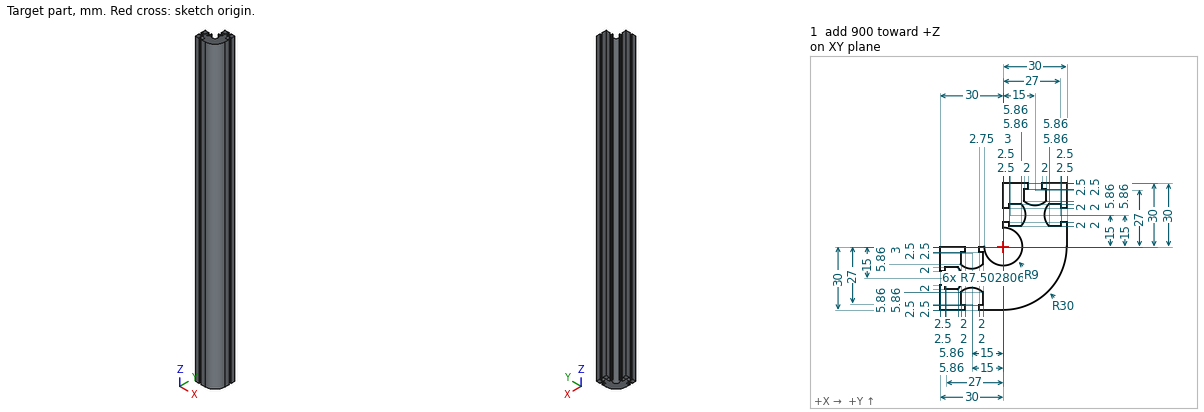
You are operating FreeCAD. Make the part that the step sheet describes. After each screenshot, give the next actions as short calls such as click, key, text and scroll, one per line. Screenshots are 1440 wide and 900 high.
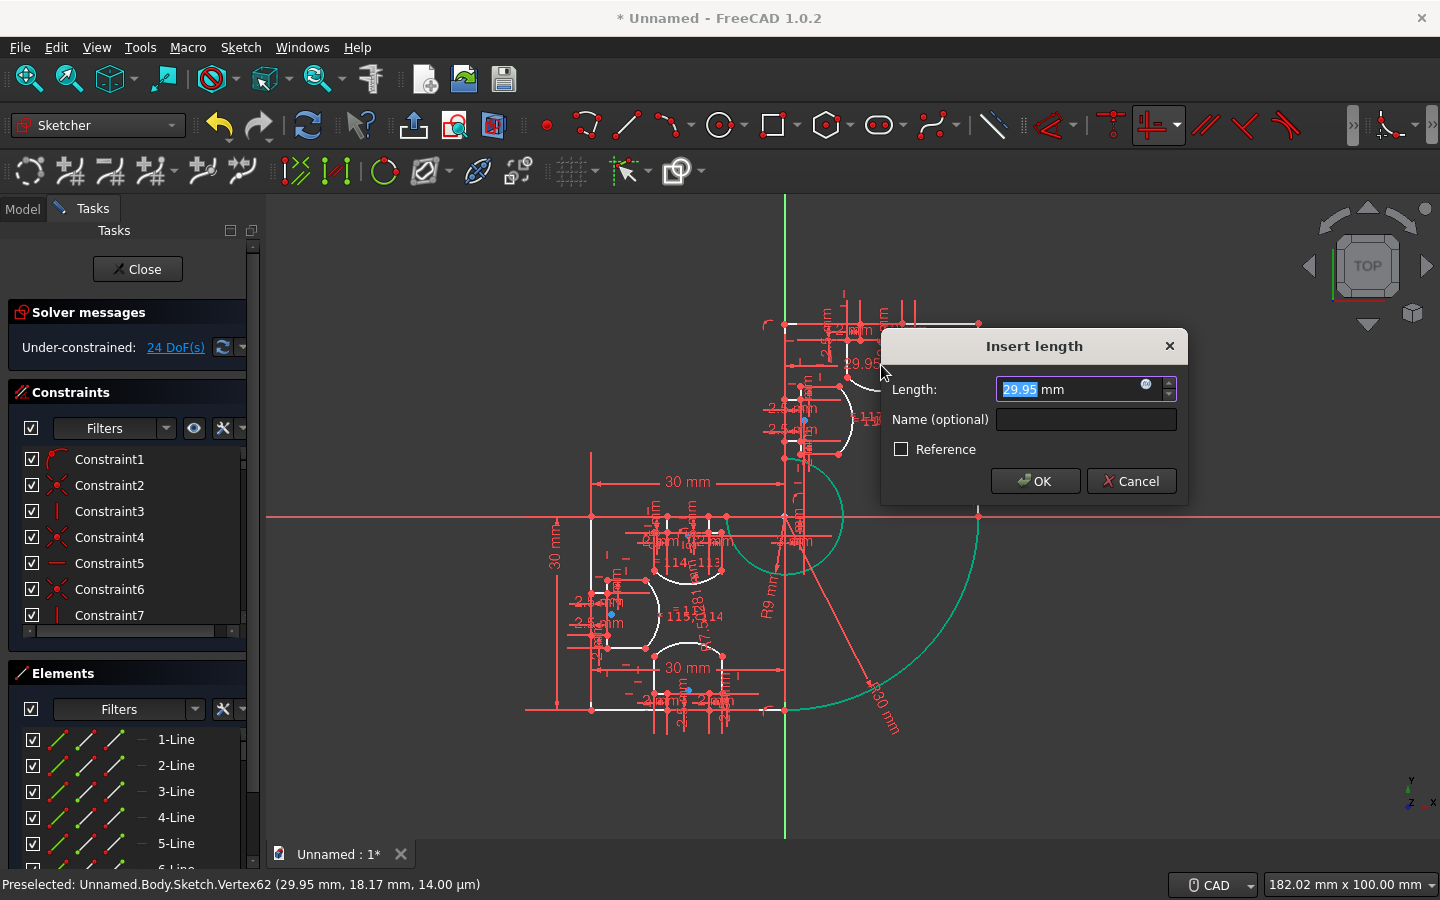
text(30)
key(Return)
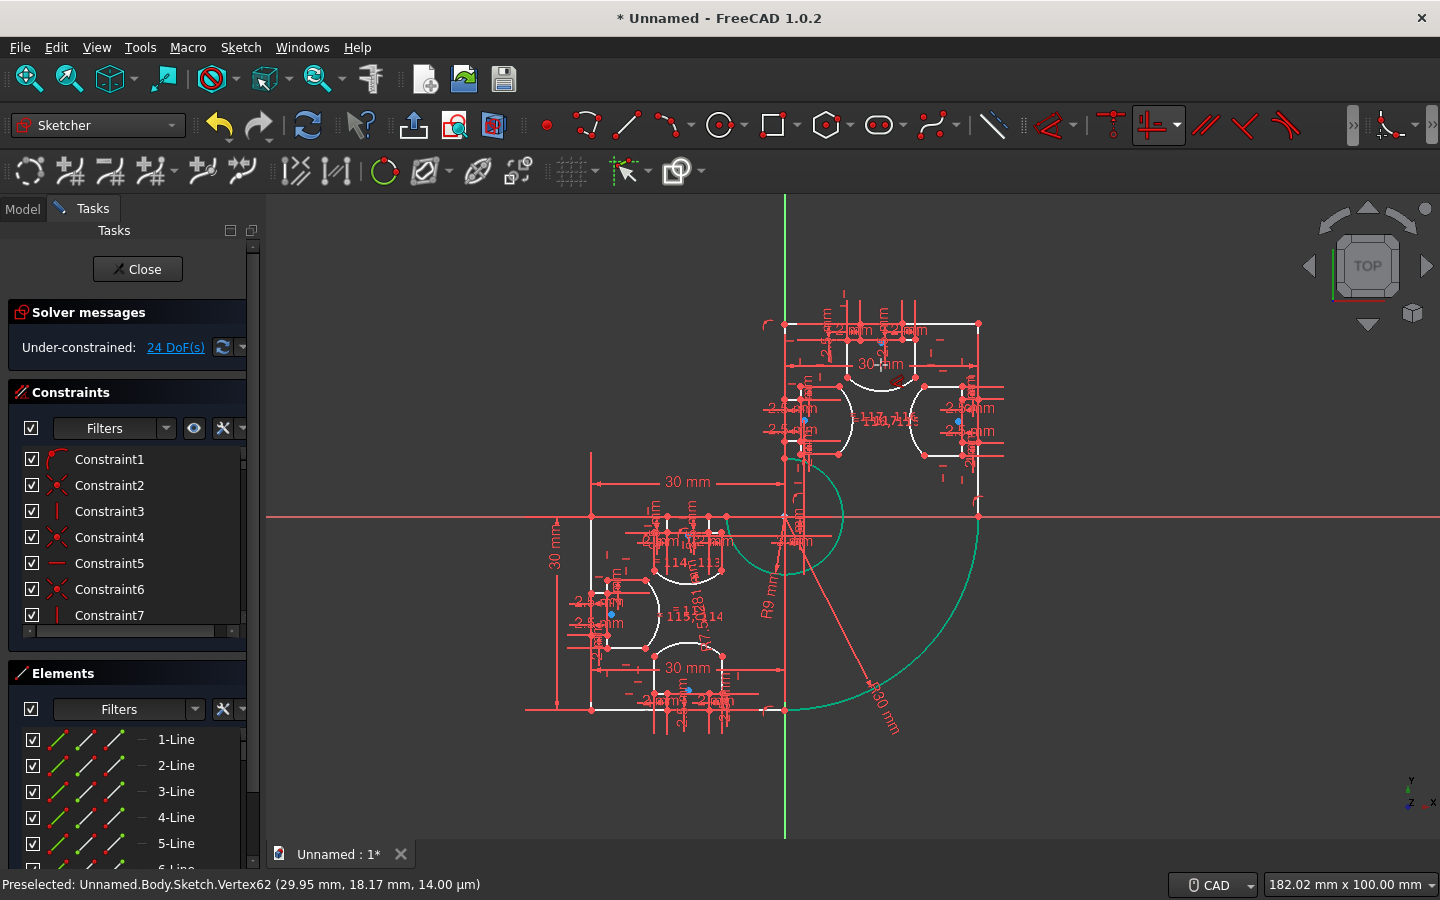
click(978, 324)
click(1012, 353)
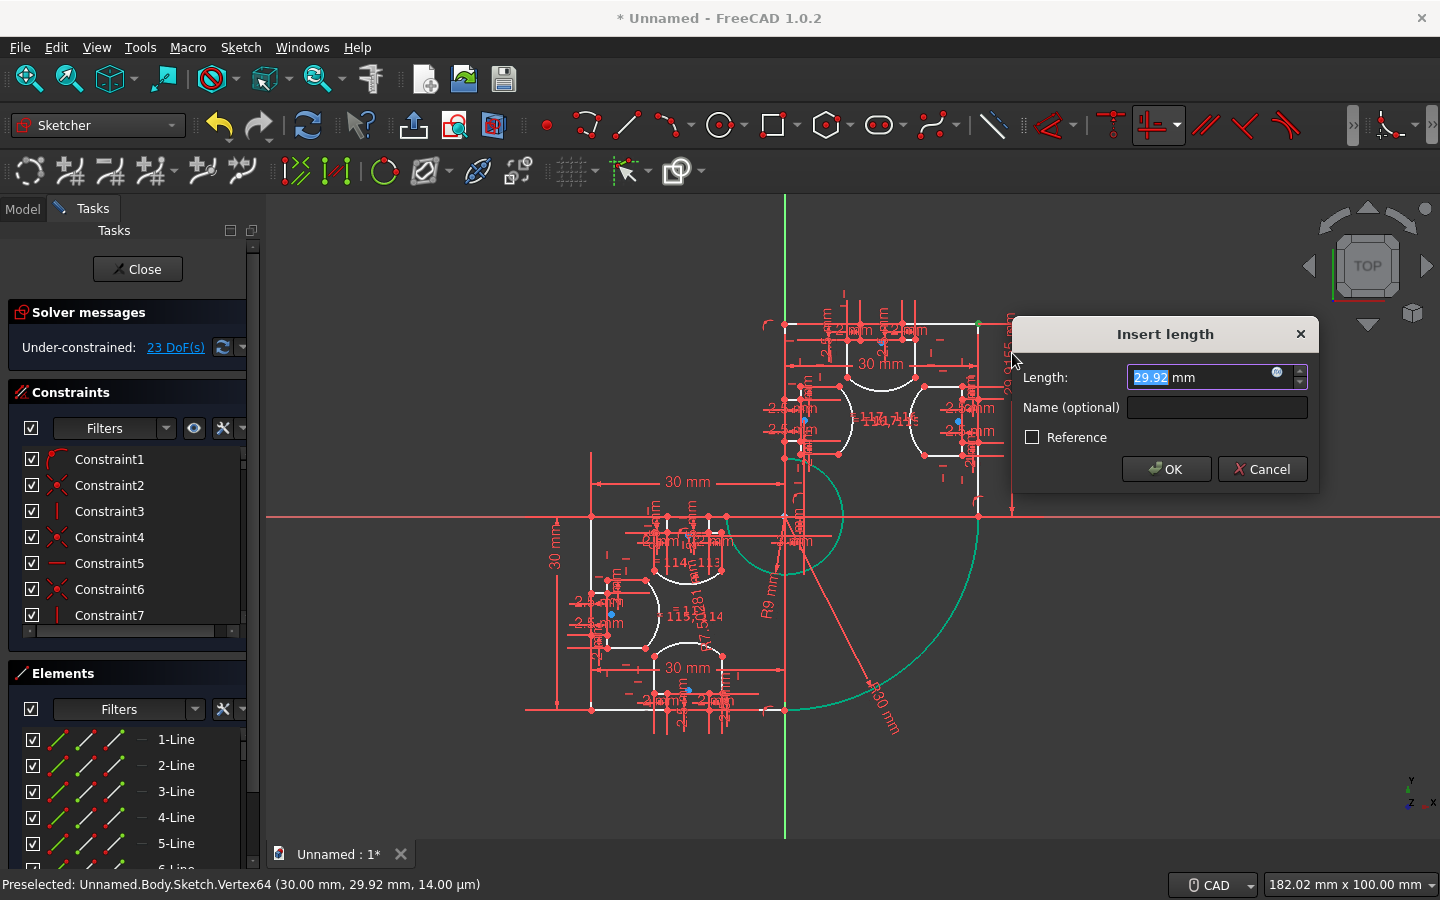
text(30)
key(Return)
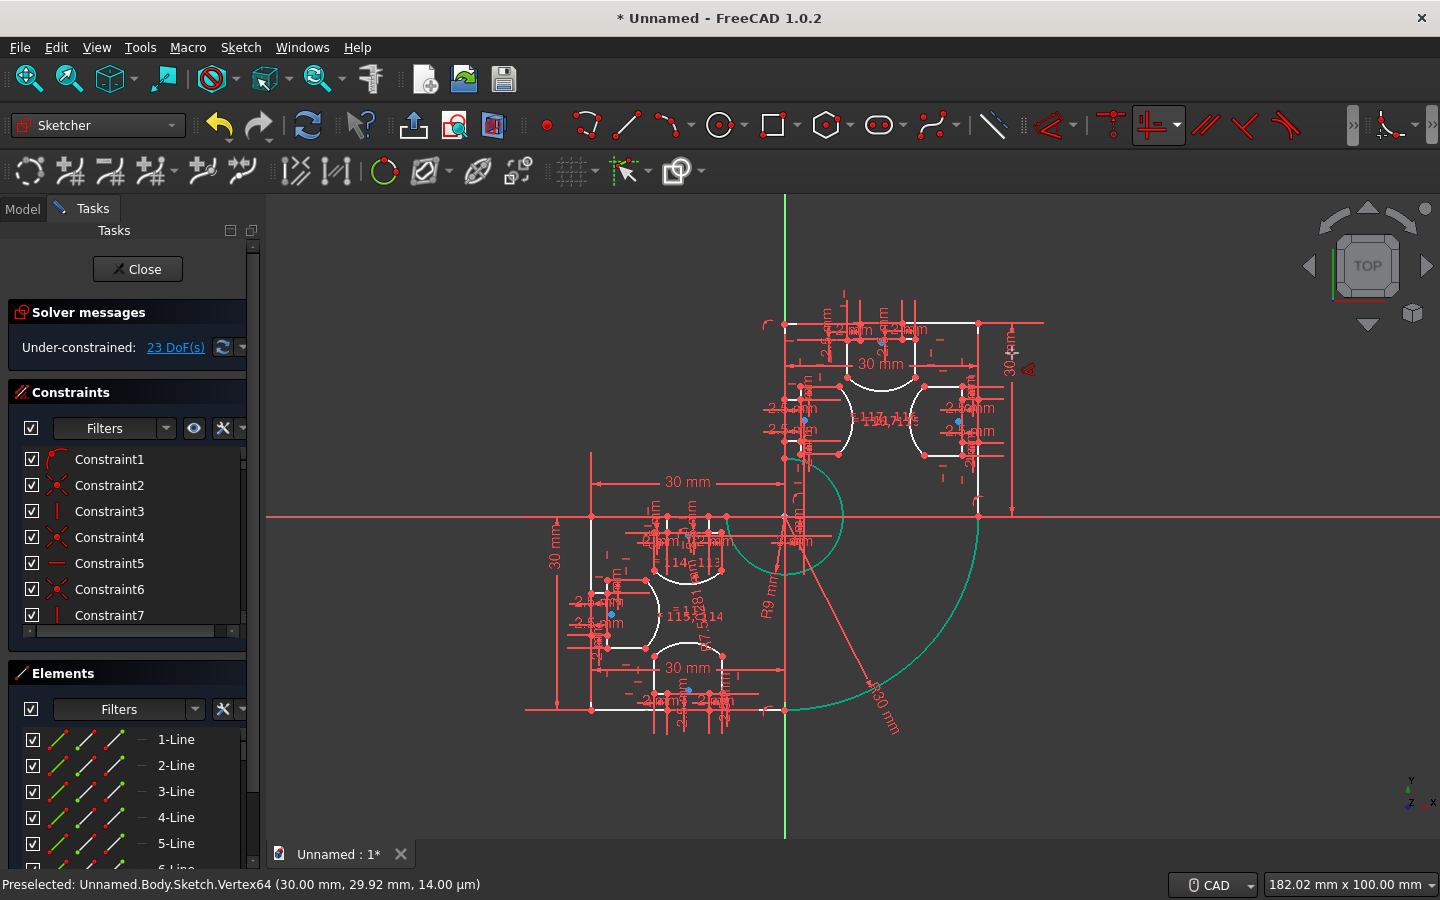
click(860, 324)
click(894, 420)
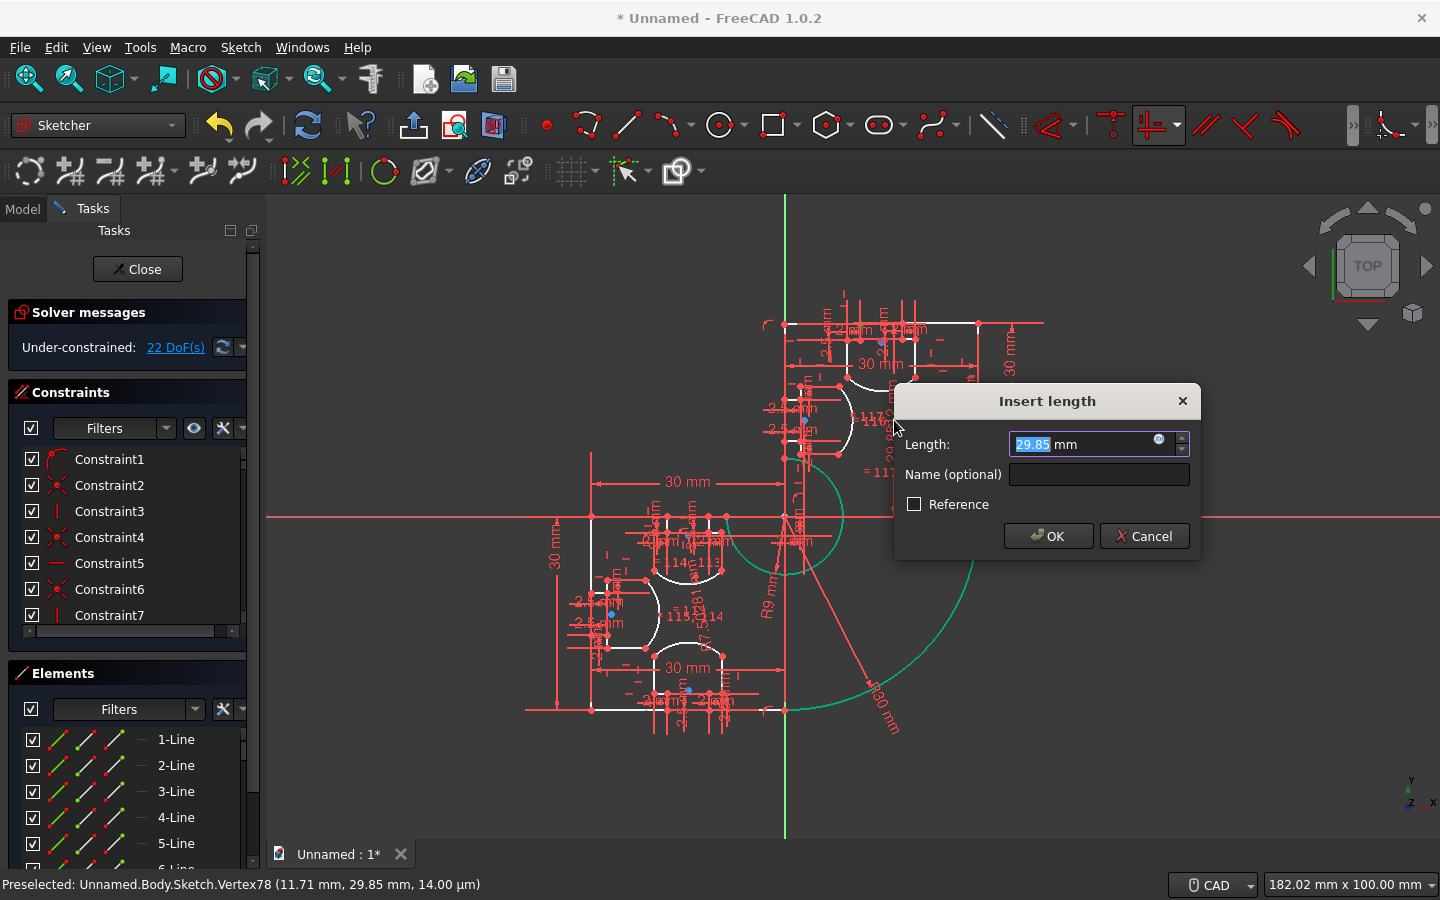
text(30)
key(Return)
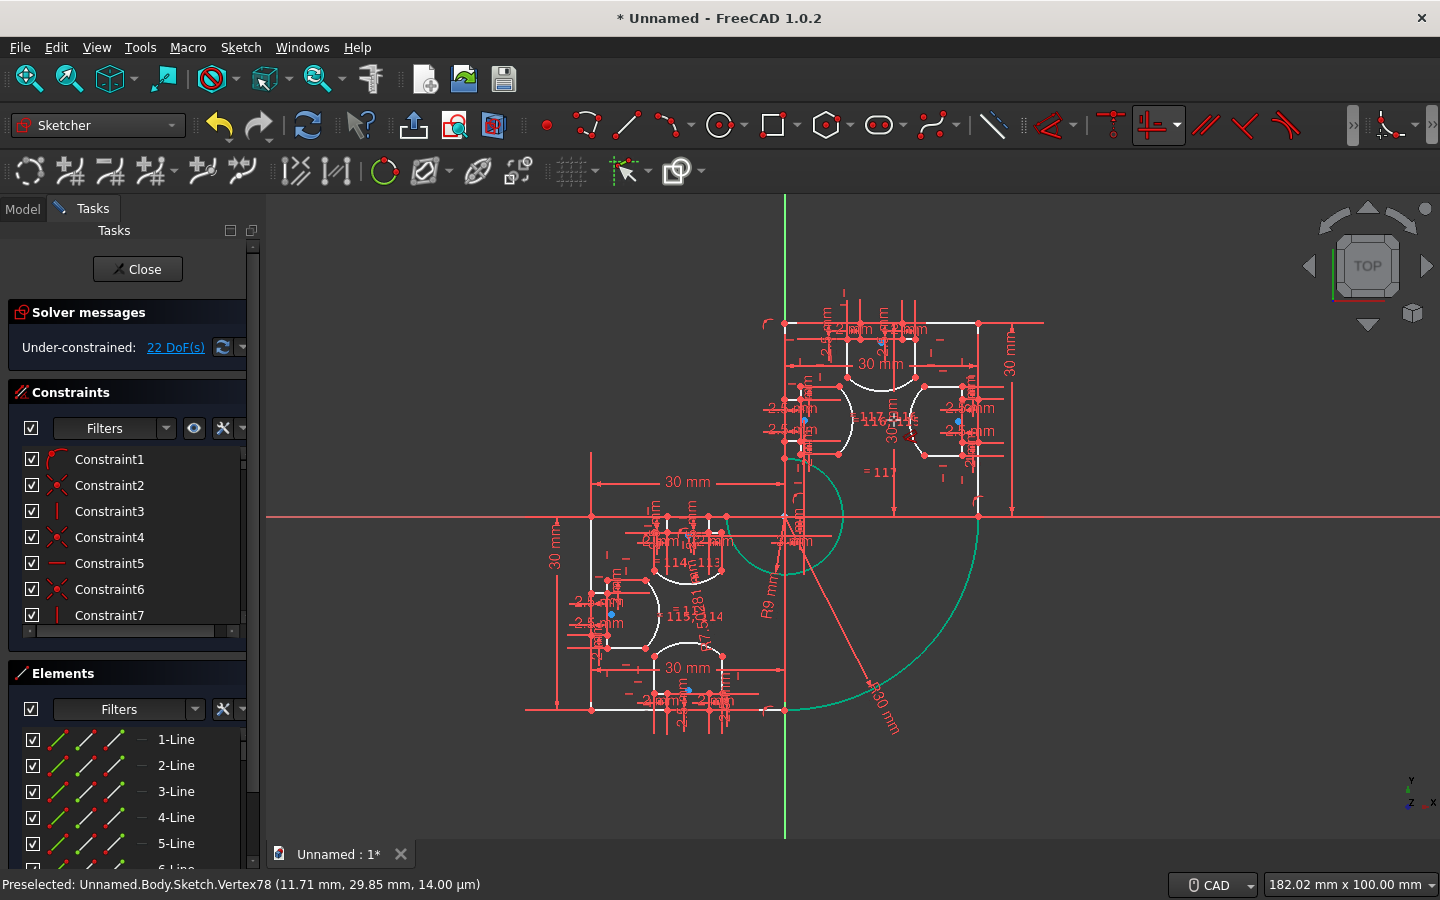
click(688, 536)
click(736, 570)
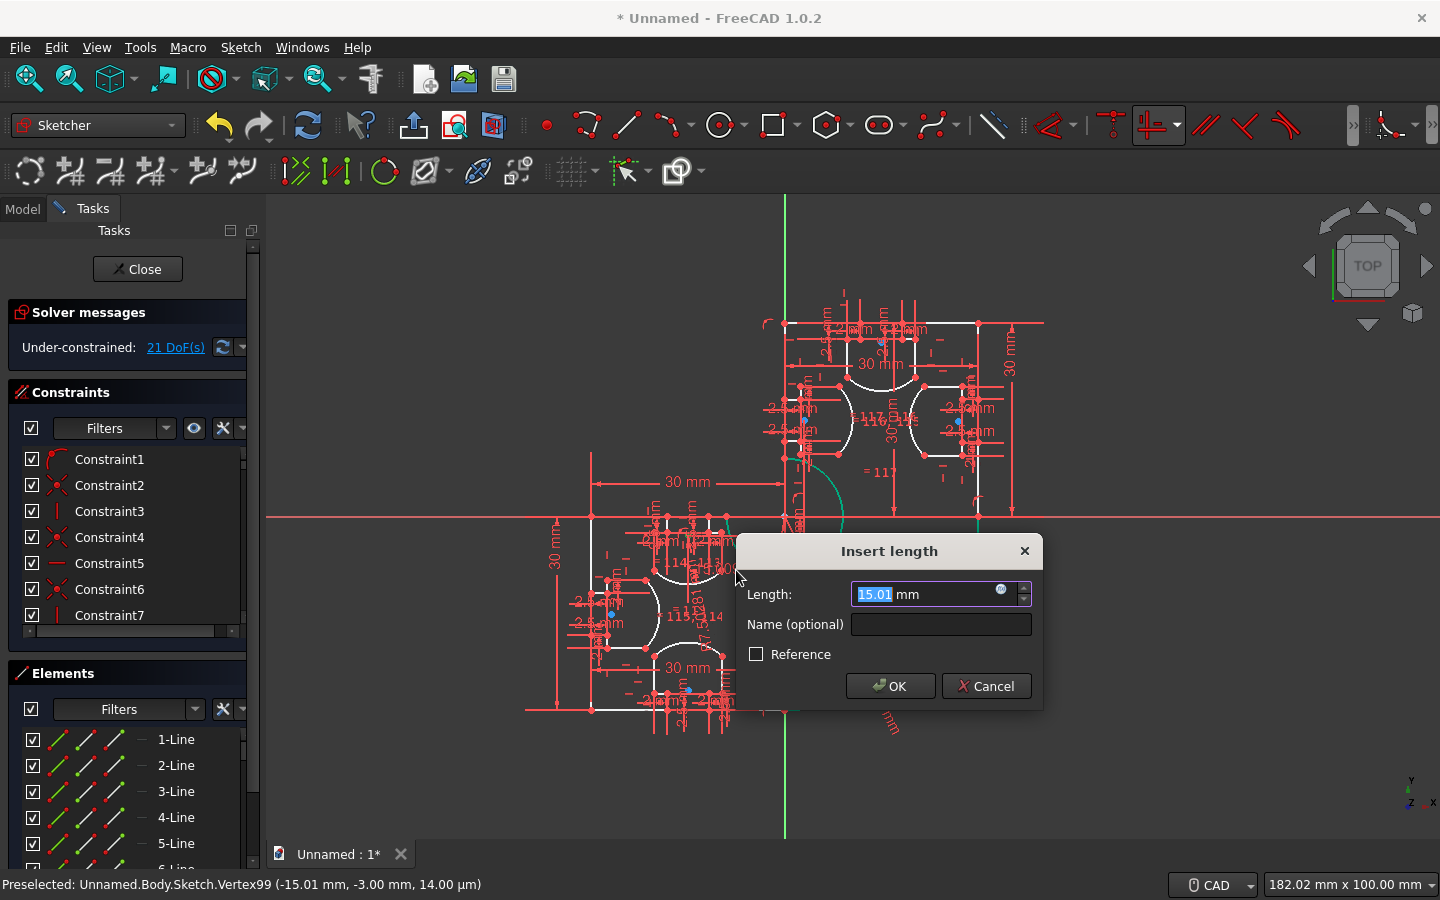
text(15)
key(Return)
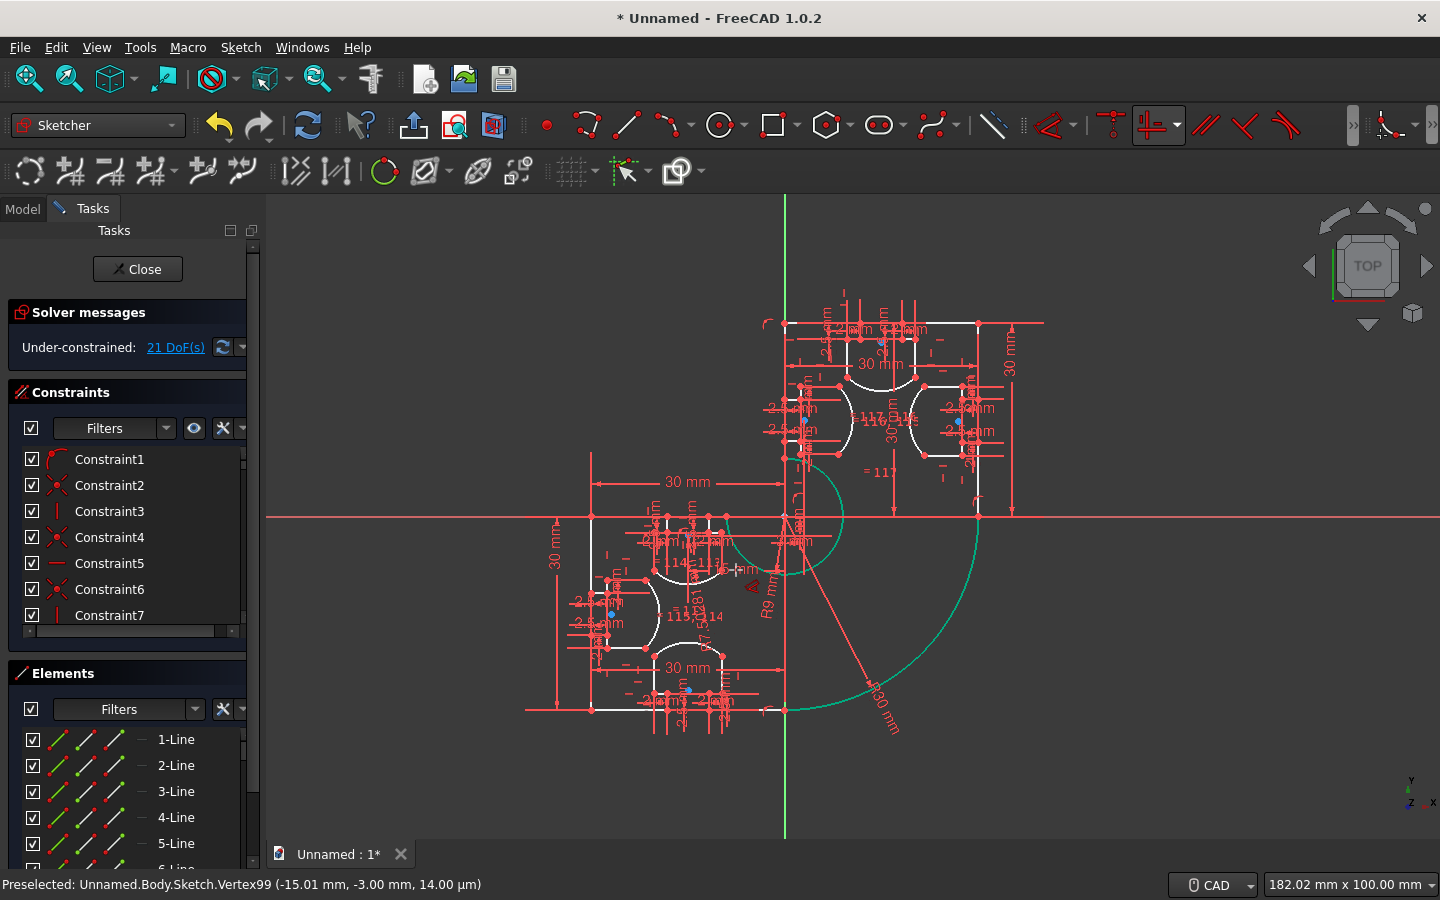
click(611, 614)
click(738, 648)